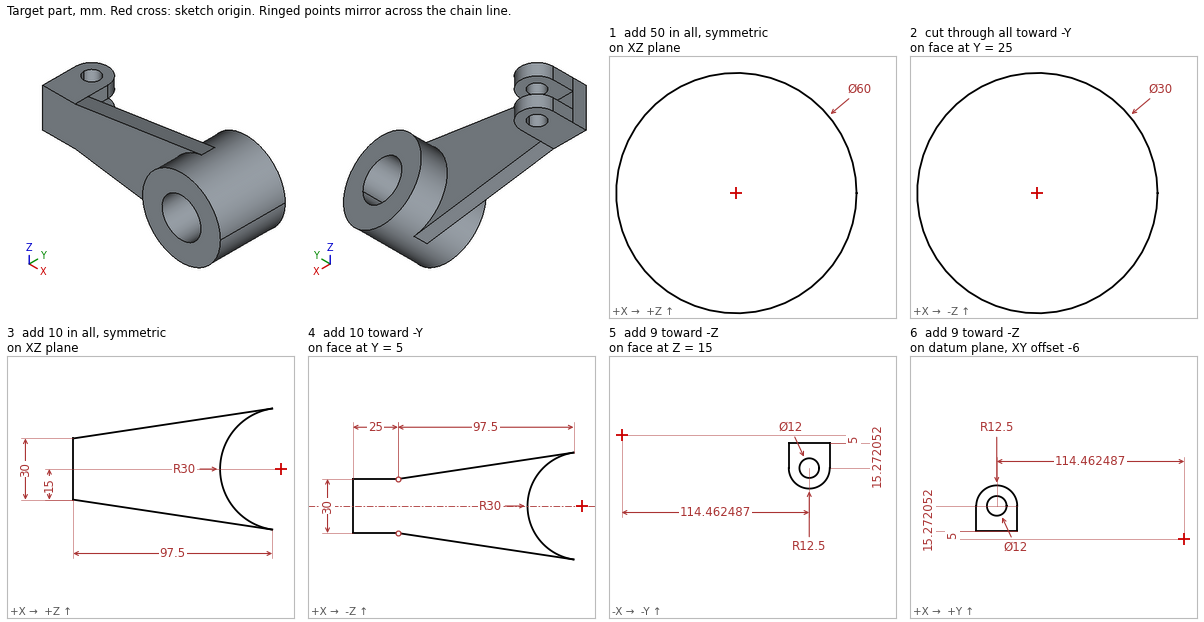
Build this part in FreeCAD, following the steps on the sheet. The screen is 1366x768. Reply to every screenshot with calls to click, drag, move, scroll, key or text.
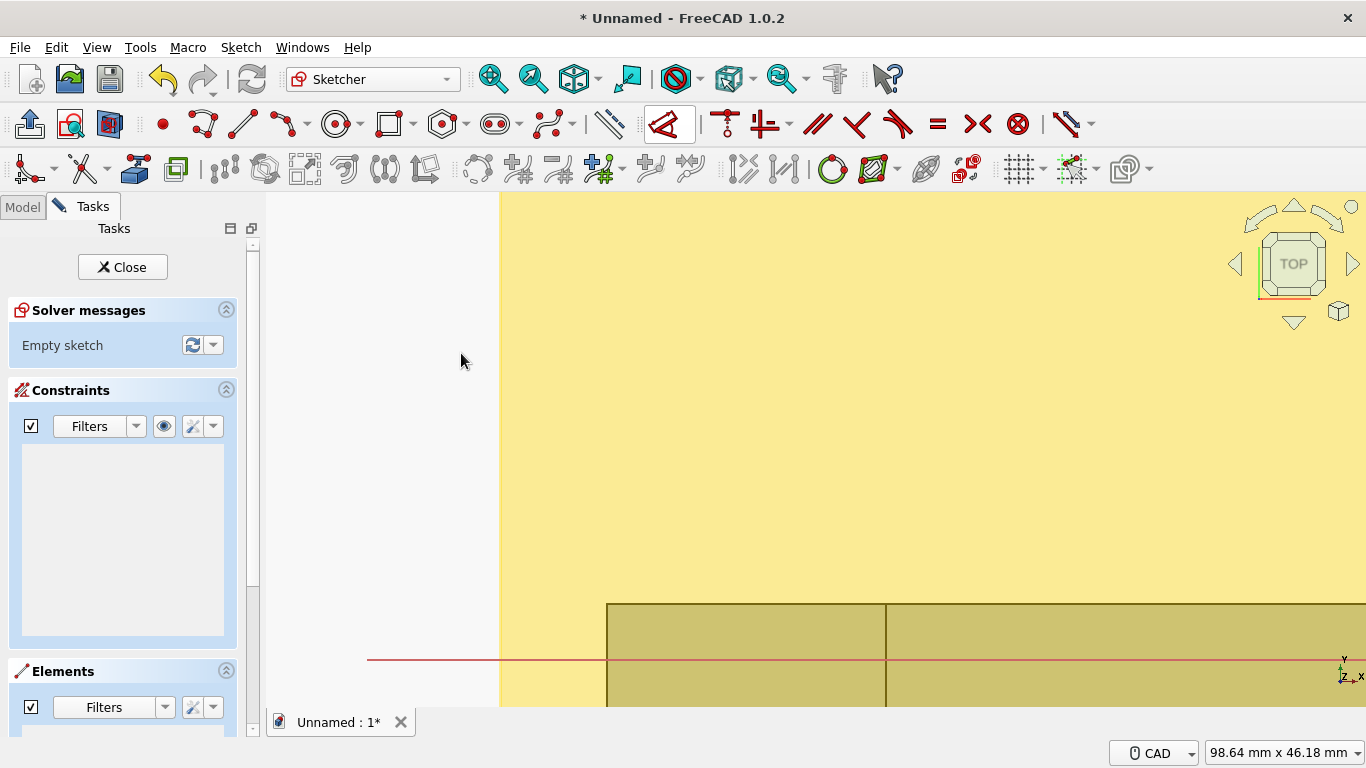
key(g)
key(m)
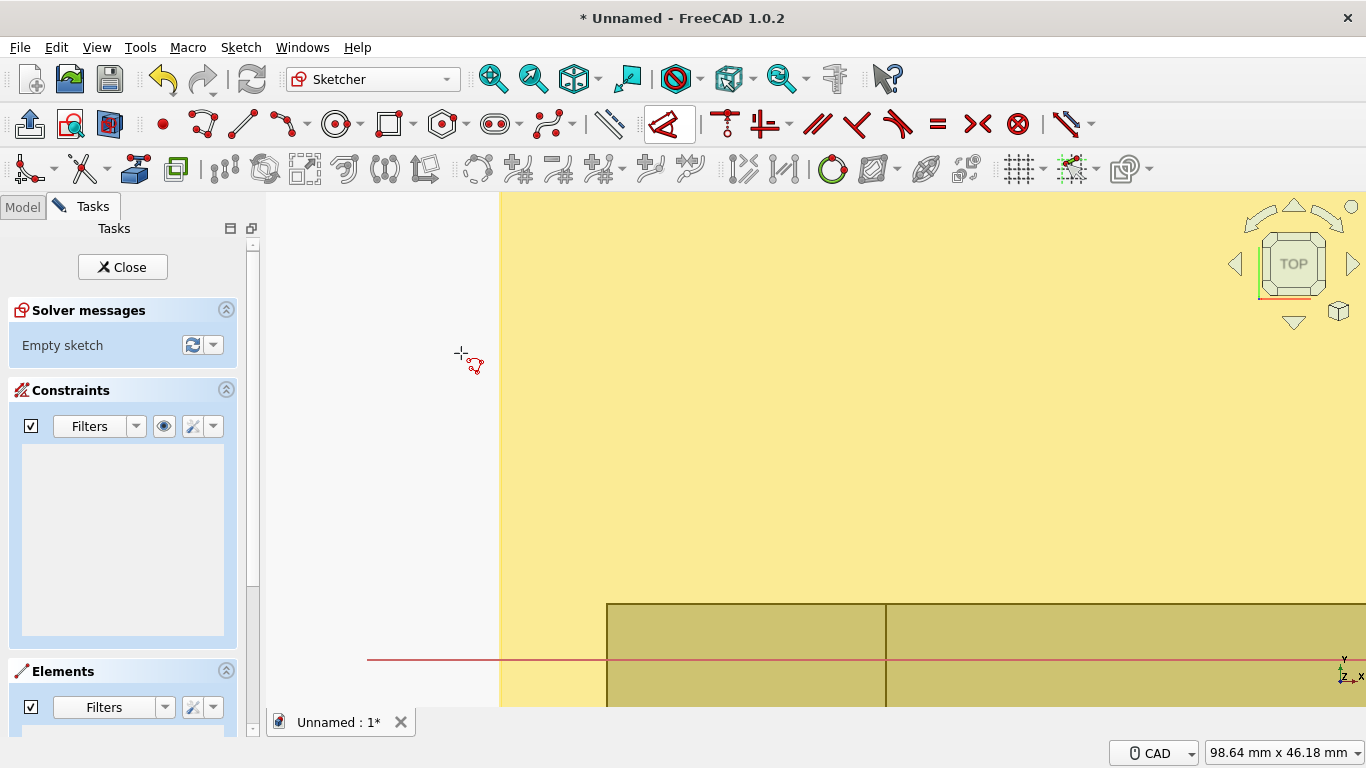
click(886, 434)
click(886, 604)
click(607, 604)
click(607, 434)
right_click(607, 434)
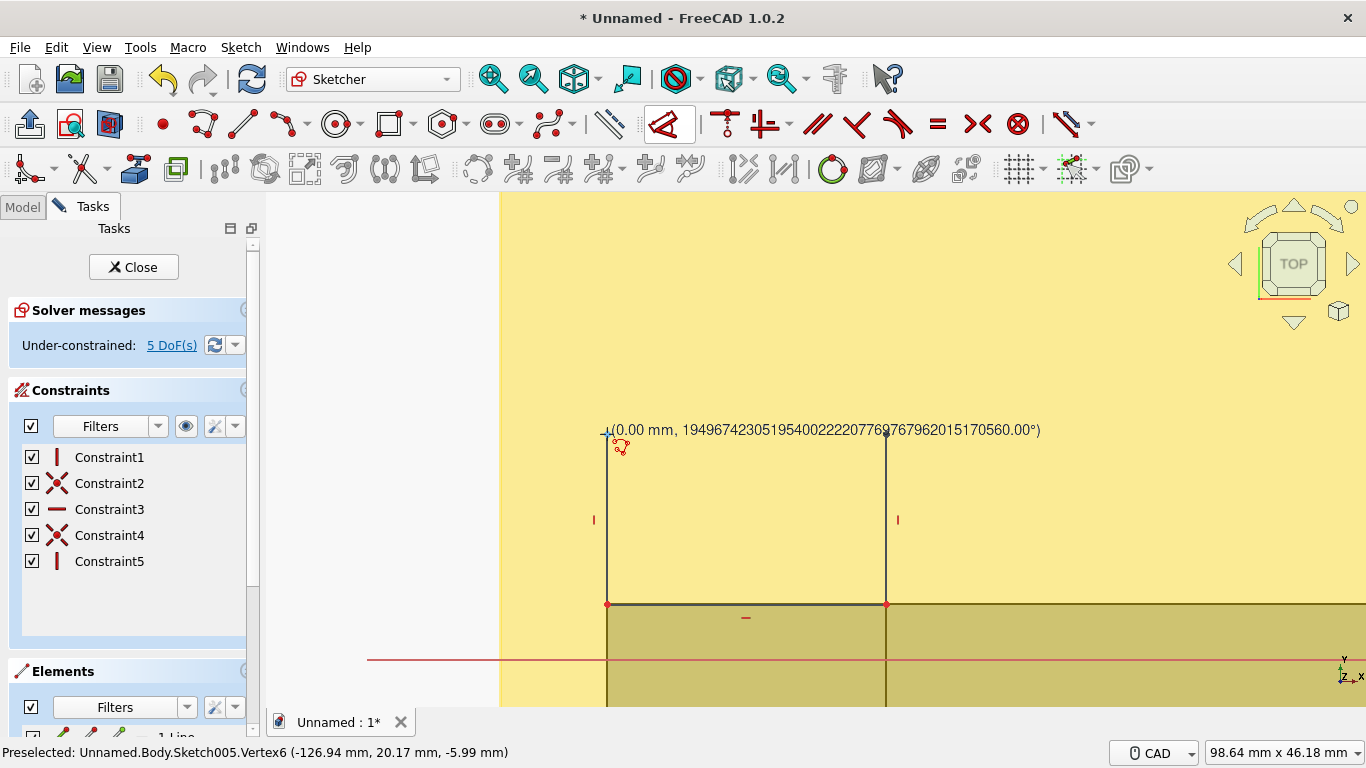
click(284, 124)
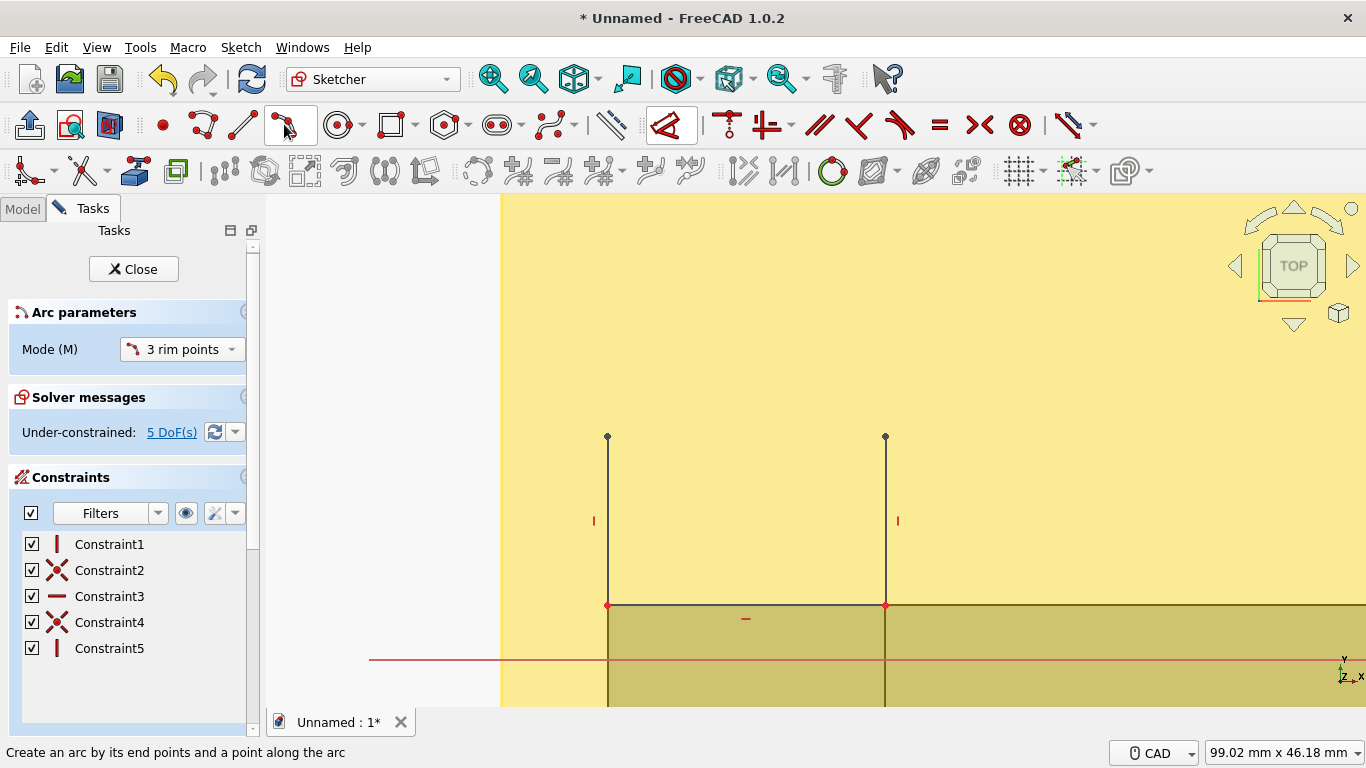
click(608, 436)
click(886, 436)
click(746, 296)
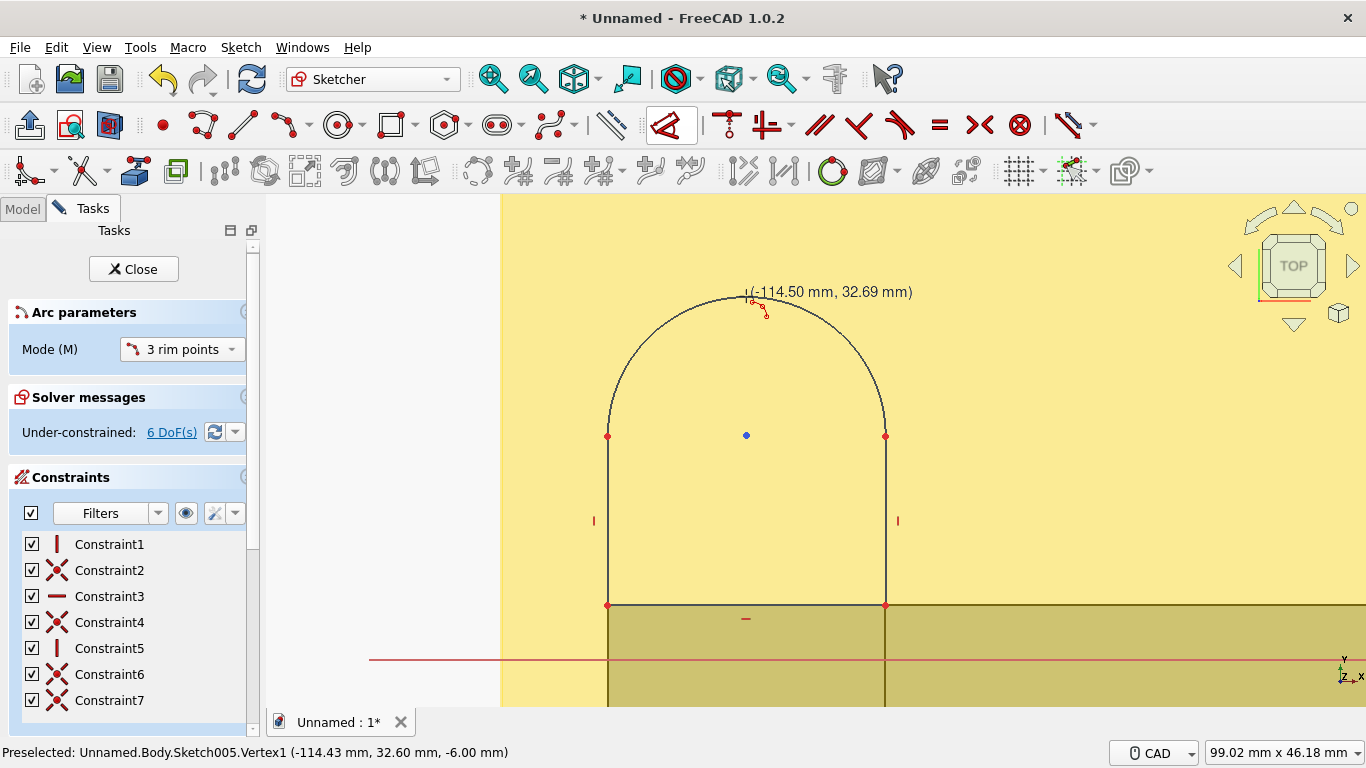
click(338, 126)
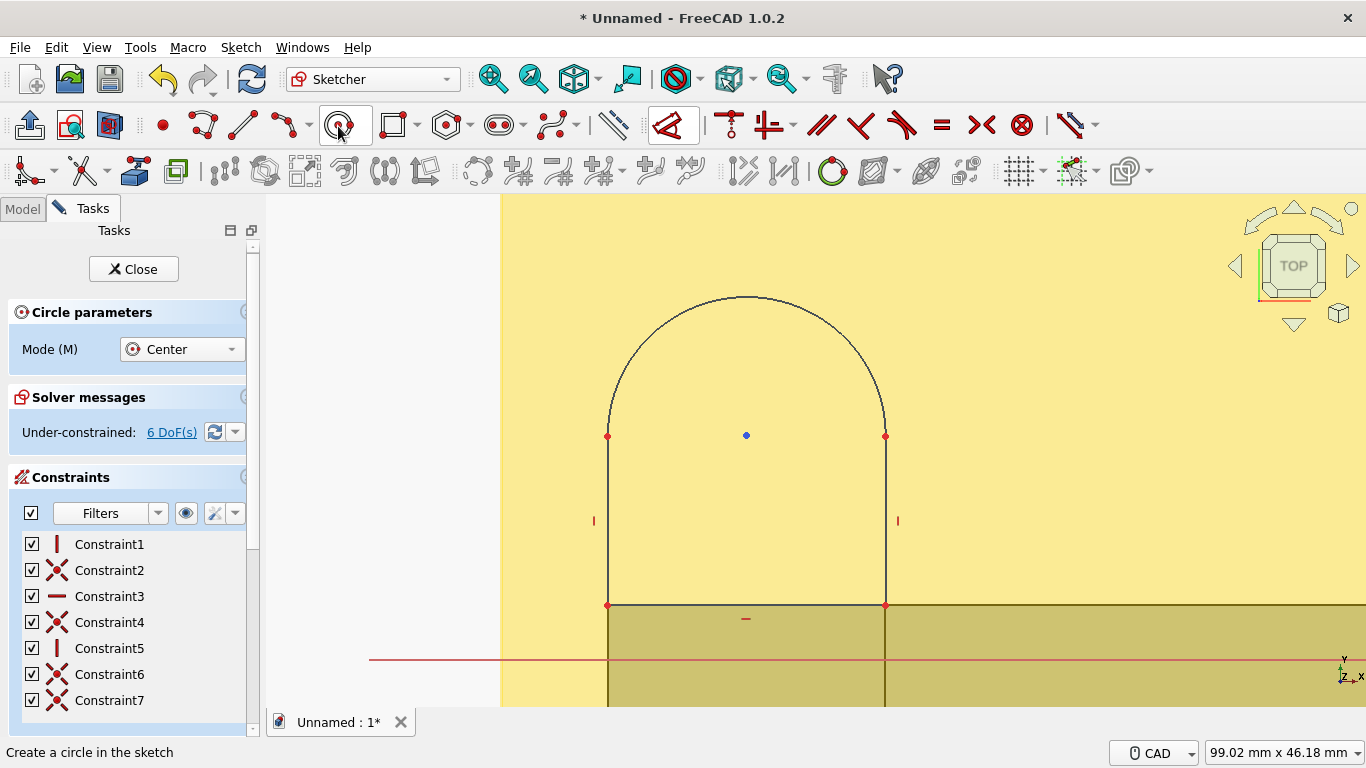
click(746, 435)
move(794, 388)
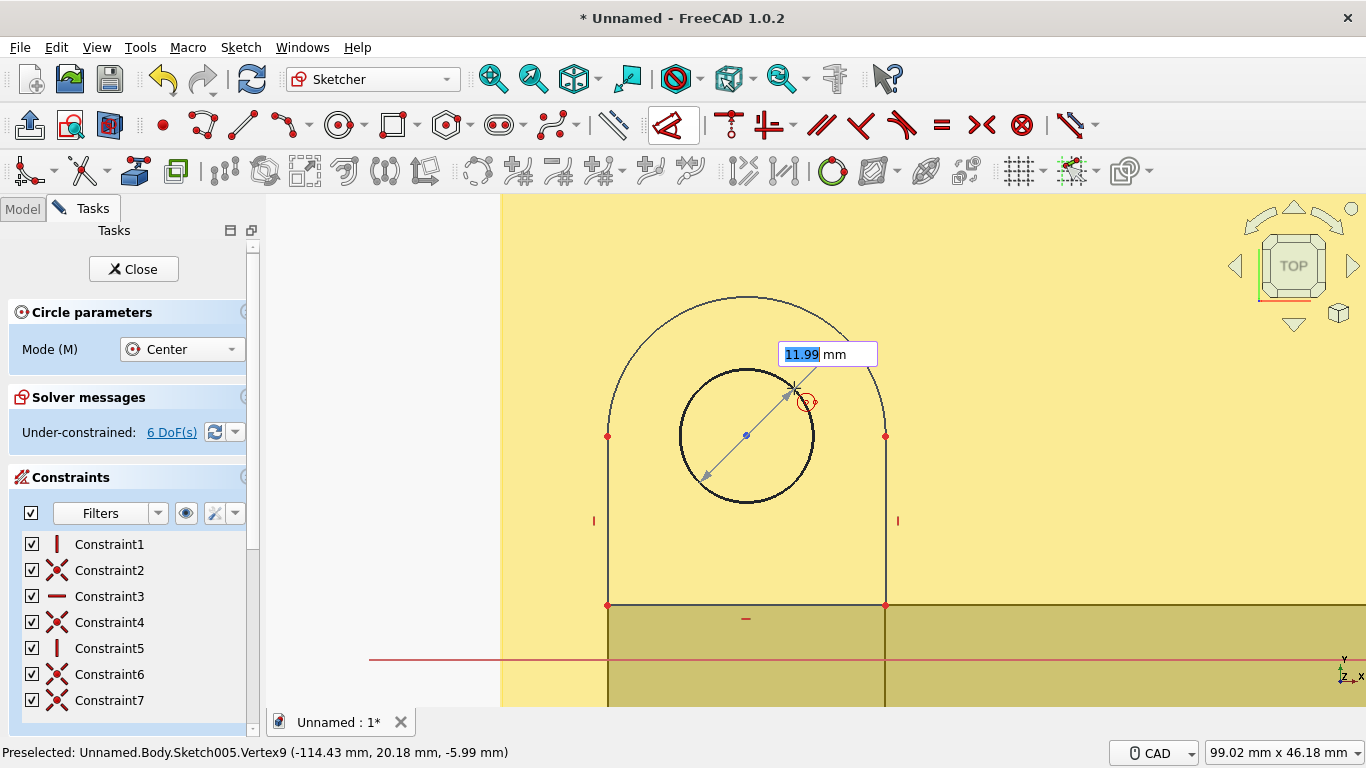
text(12)
key(Return)
key(Escape)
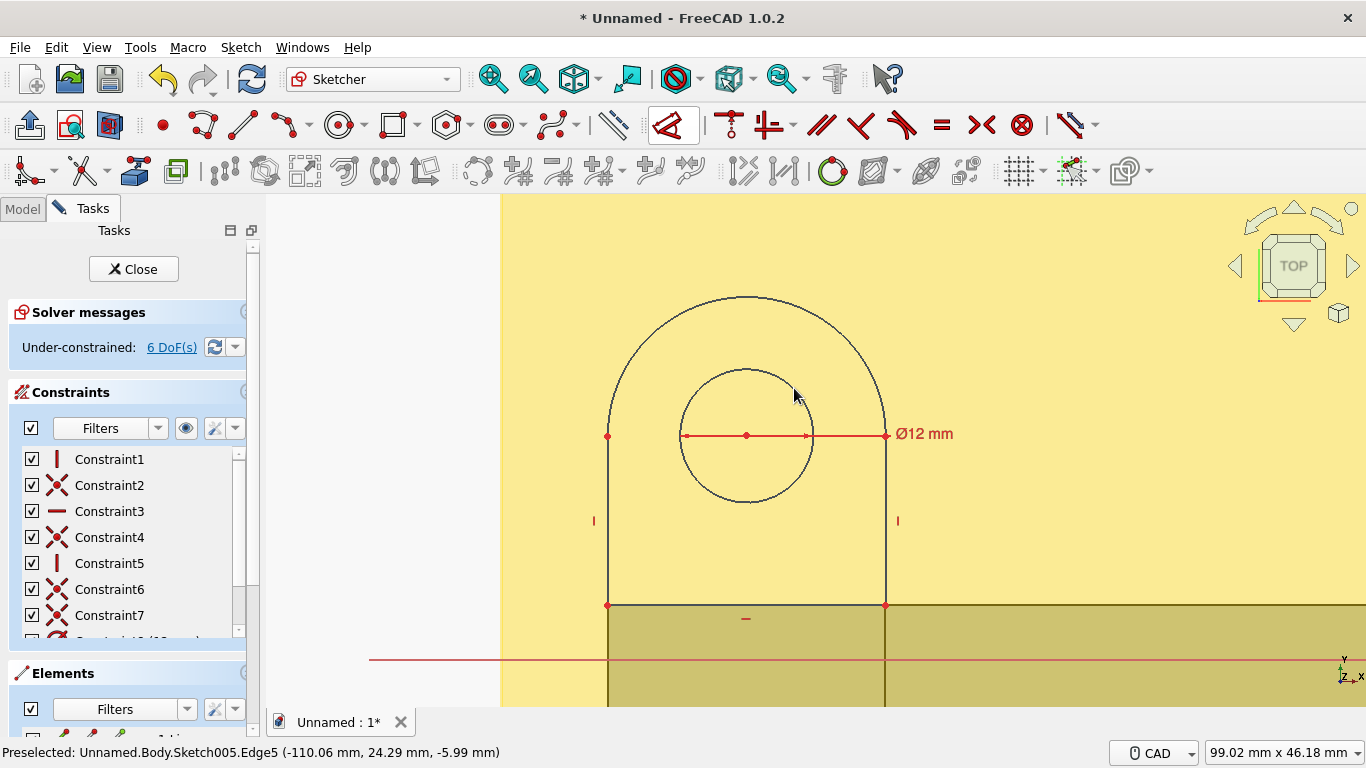
click(886, 487)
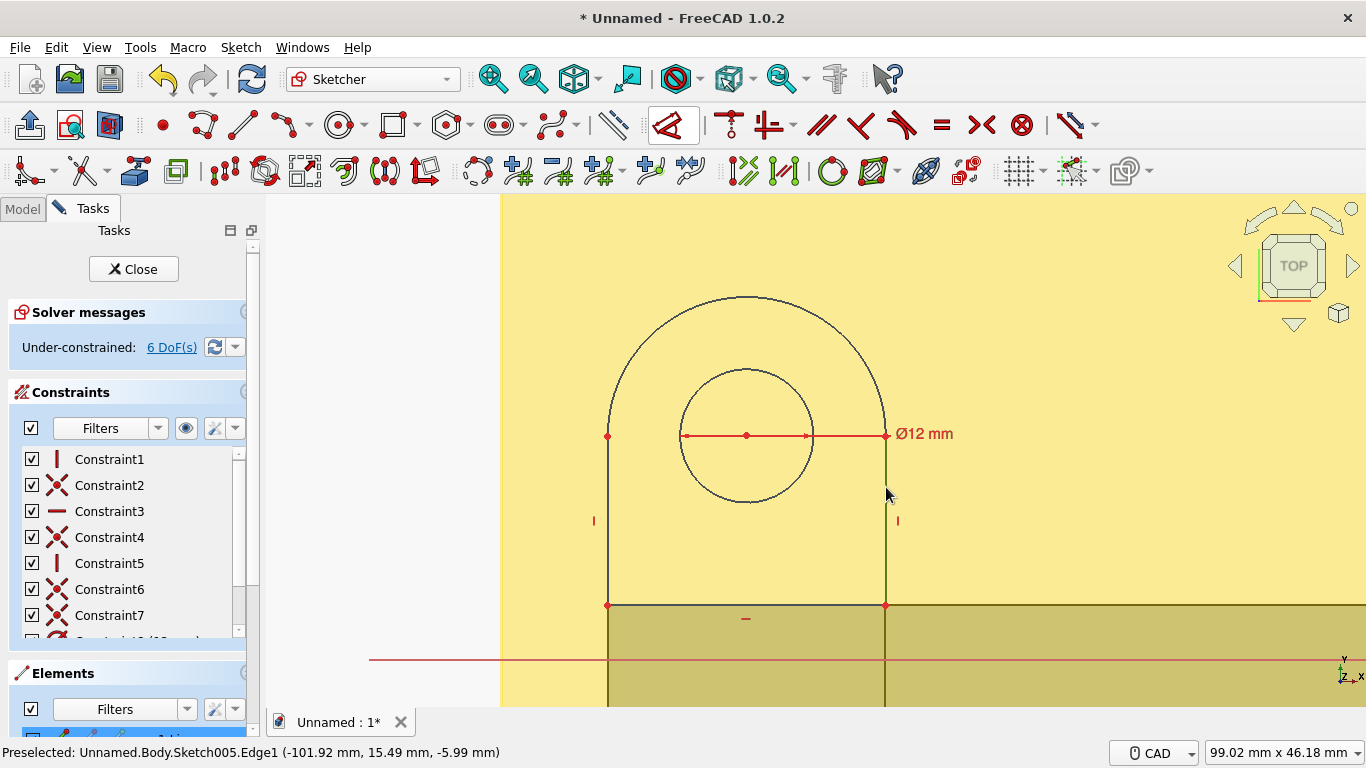
click(828, 324)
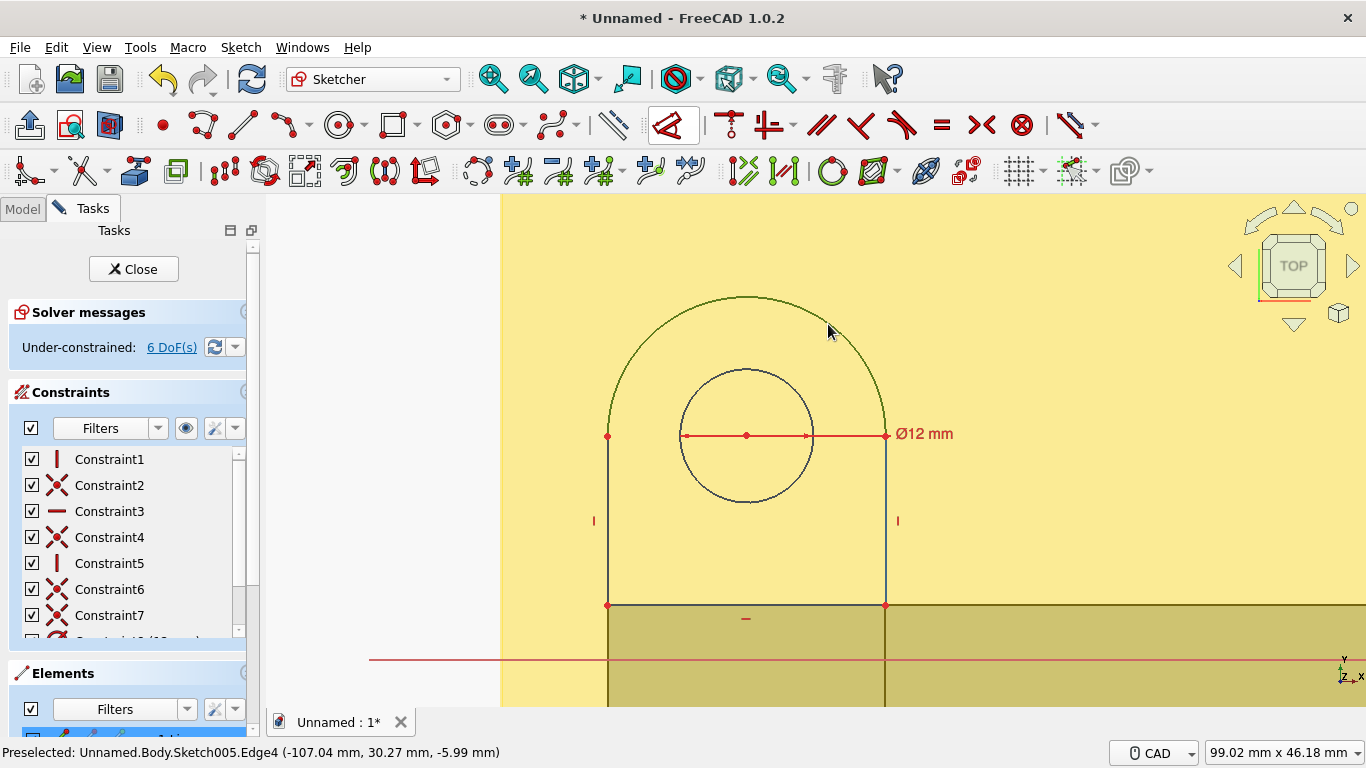
click(902, 126)